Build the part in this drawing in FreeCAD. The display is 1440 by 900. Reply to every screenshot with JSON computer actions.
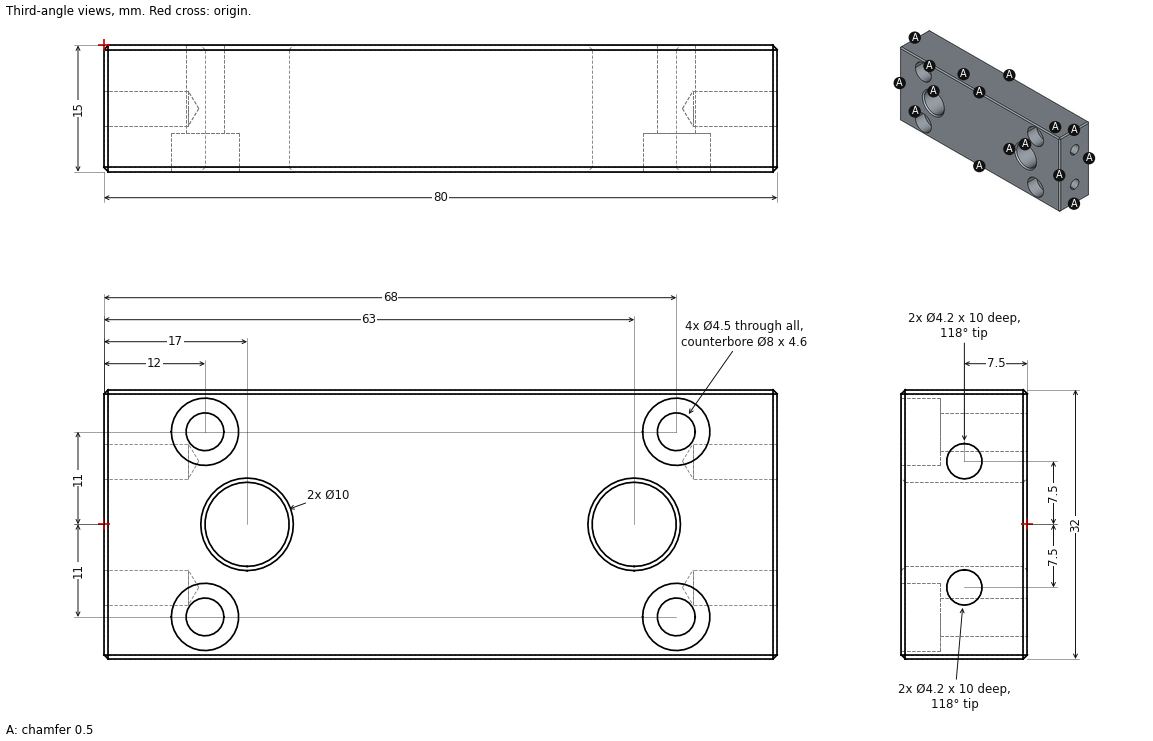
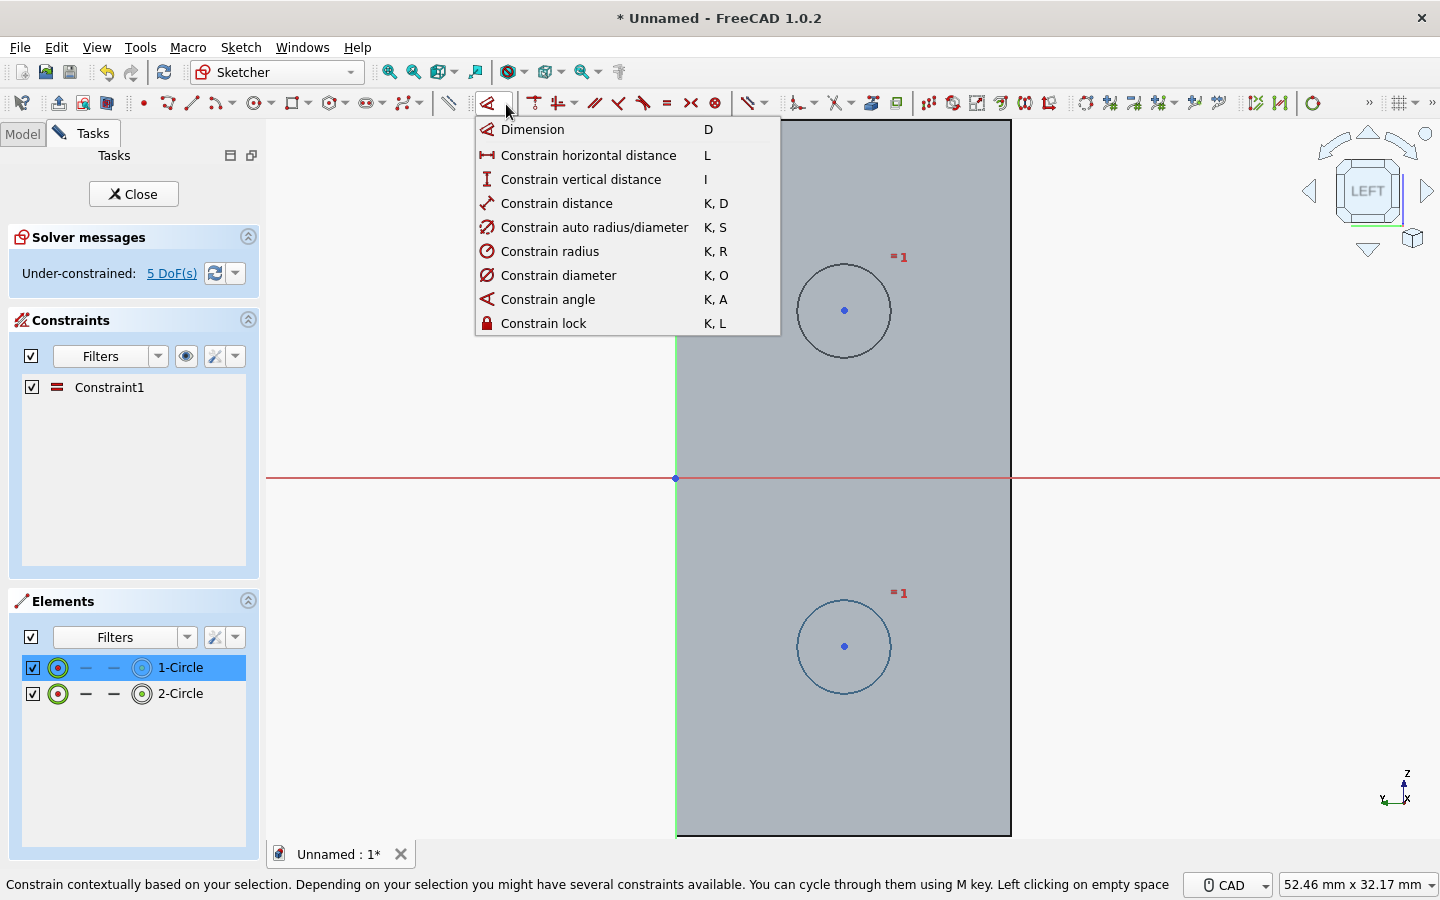
{"action": "left_click", "coordinate": [628, 275]}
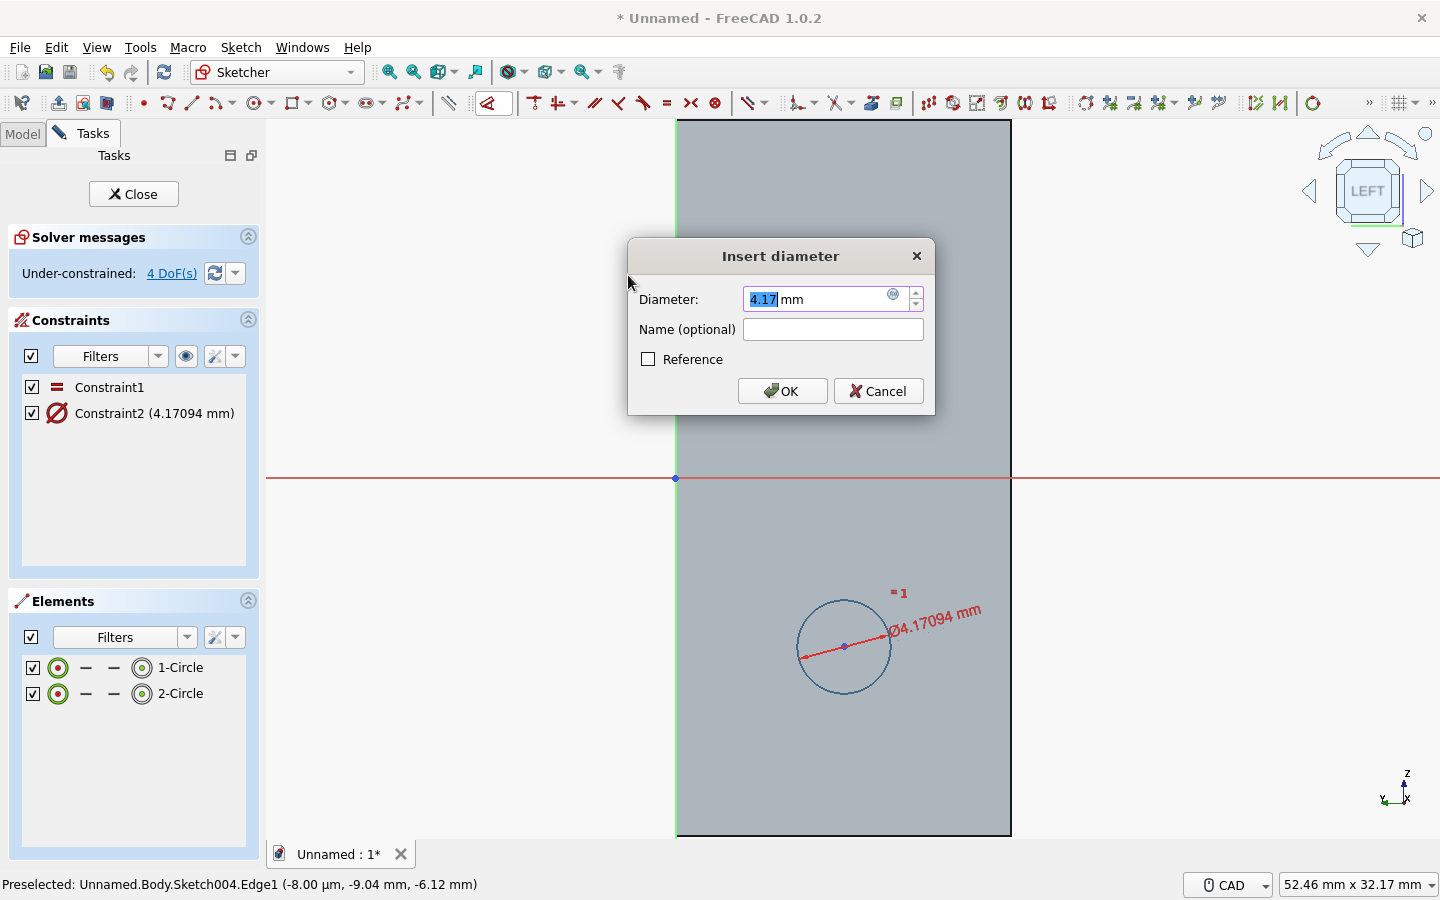
{"action": "type", "text": "4.2"}
{"action": "key", "text": "Return"}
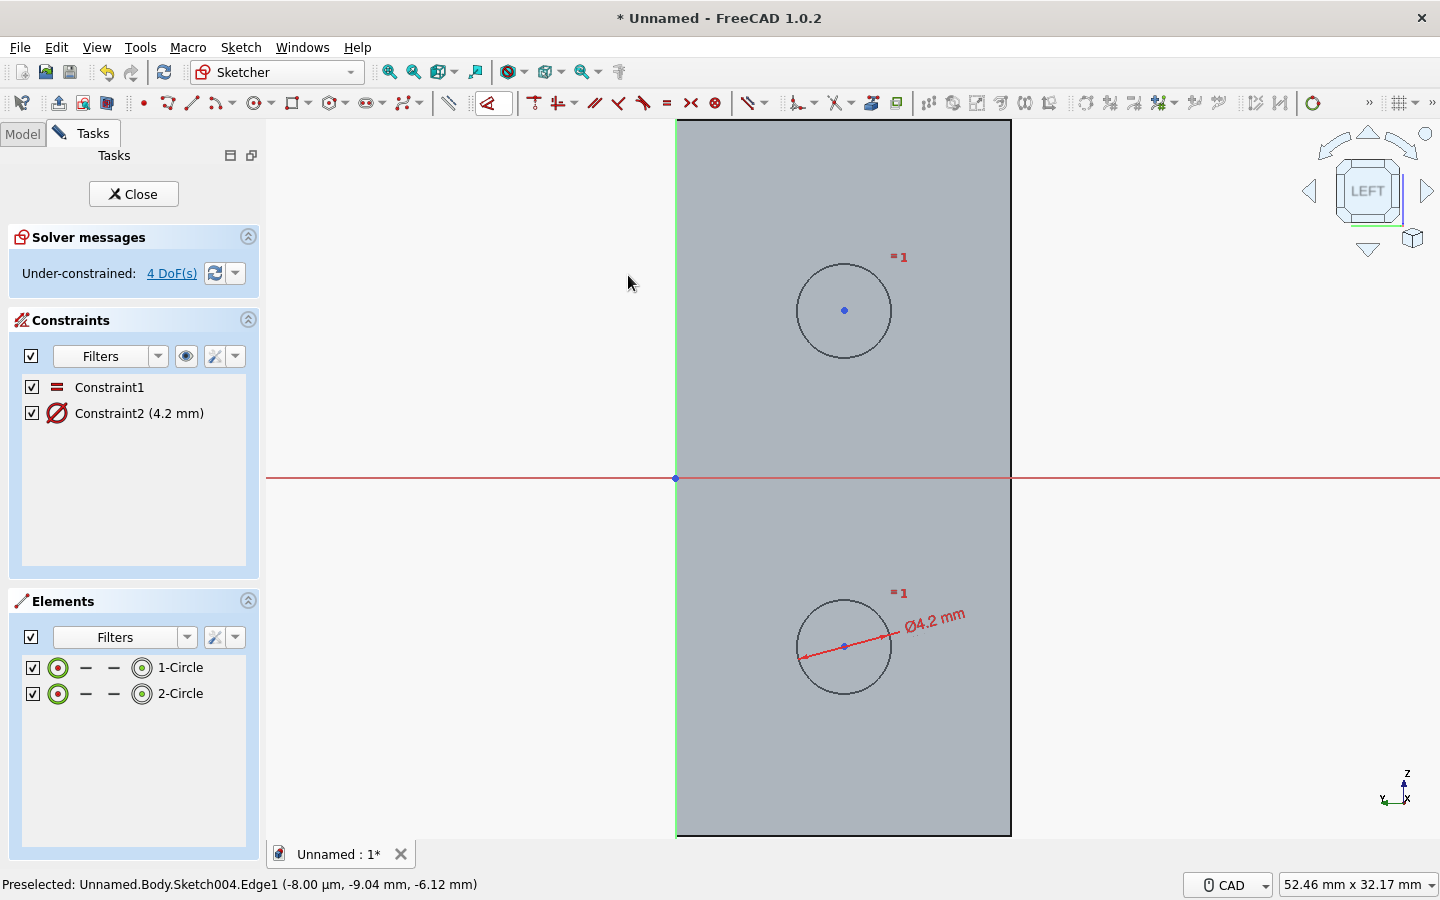
{"action": "left_click", "coordinate": [844, 647]}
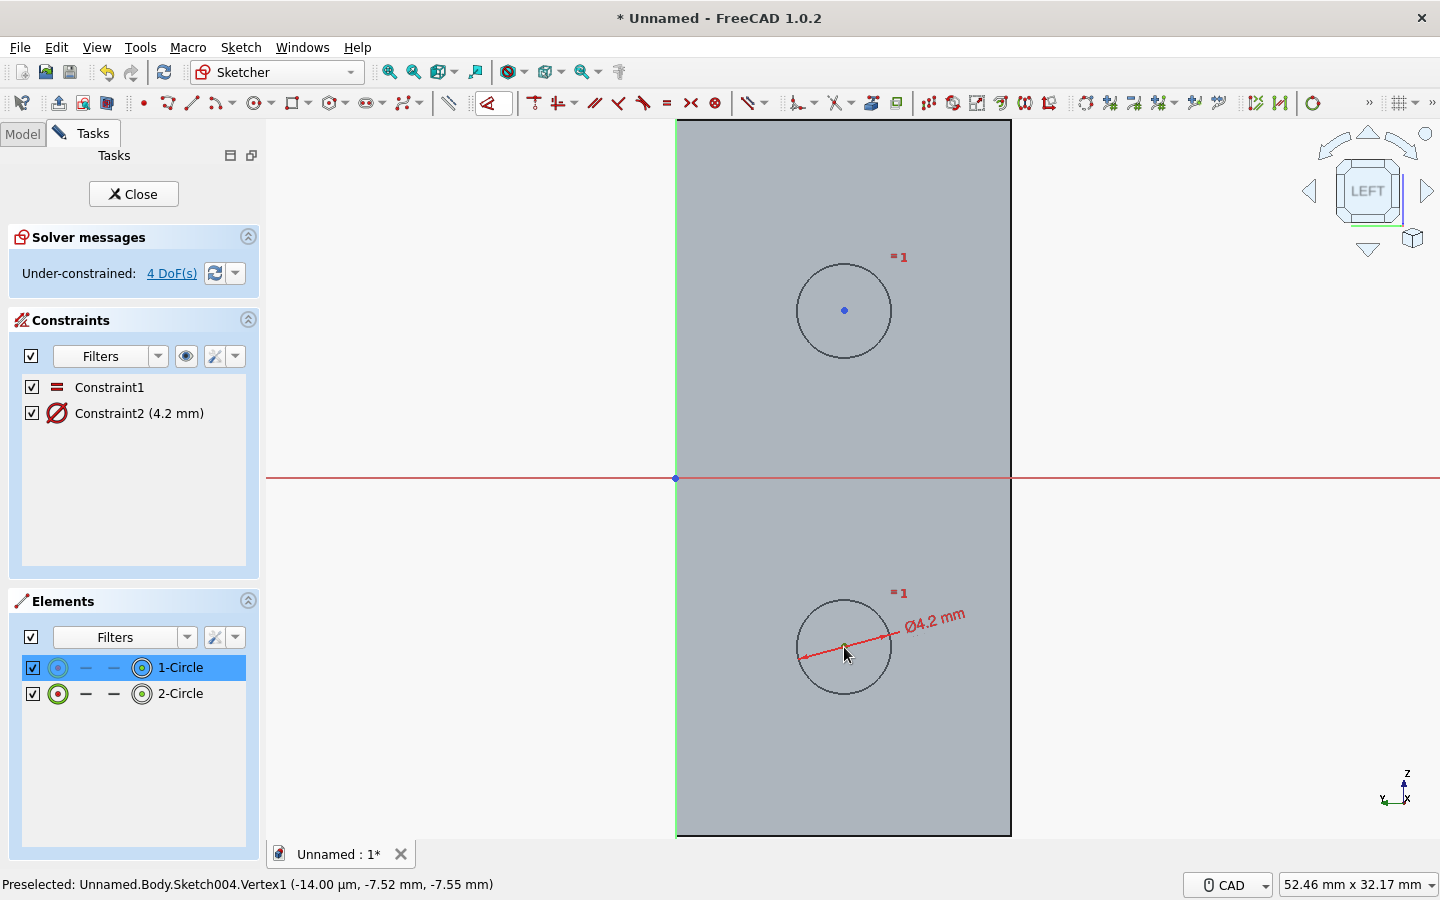
{"action": "left_click", "coordinate": [506, 104]}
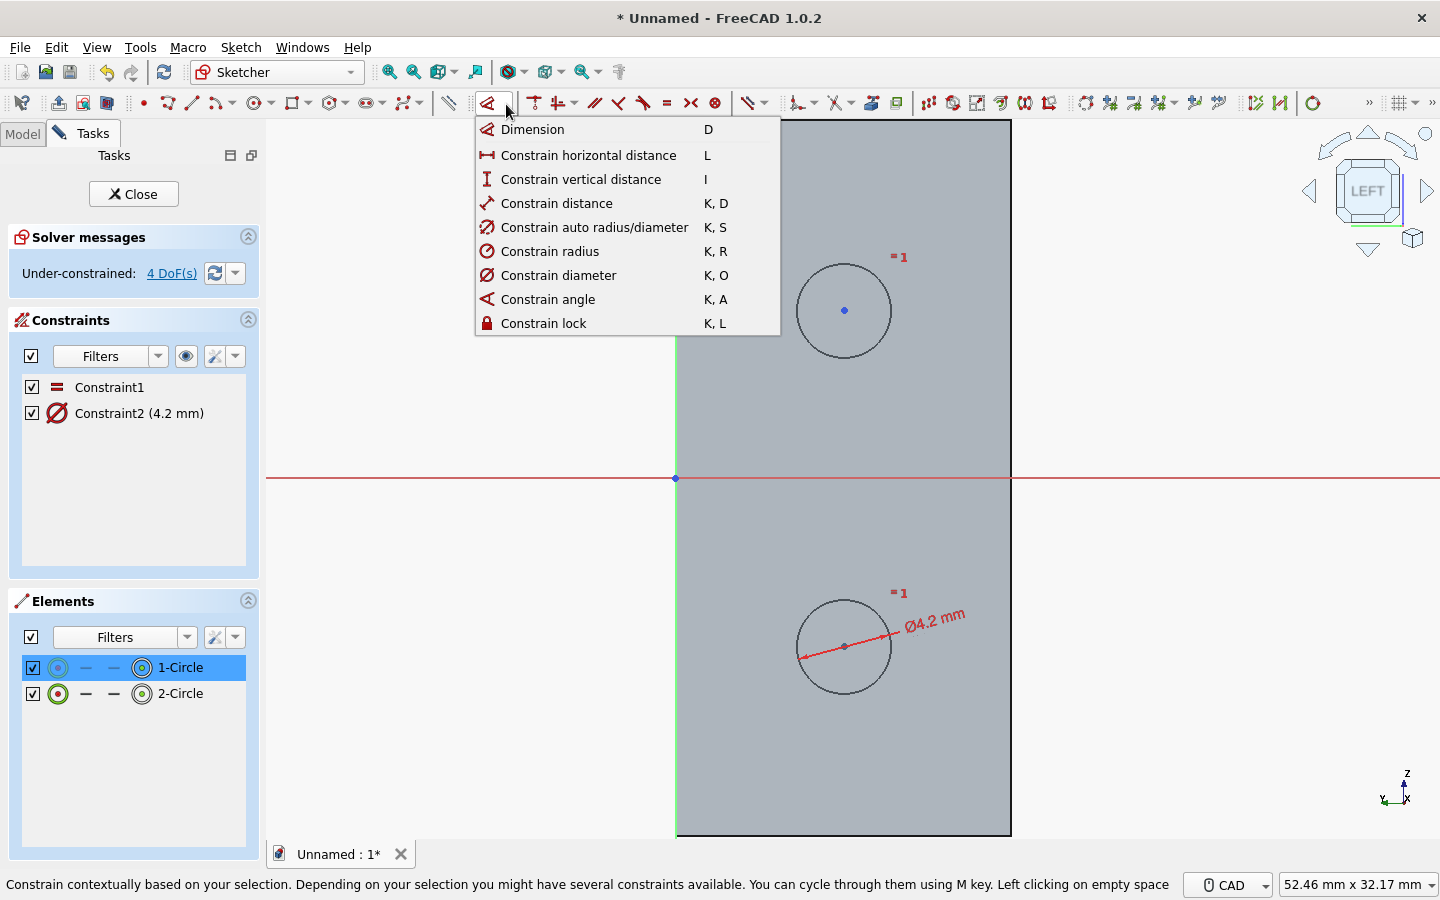
{"action": "left_click", "coordinate": [628, 155]}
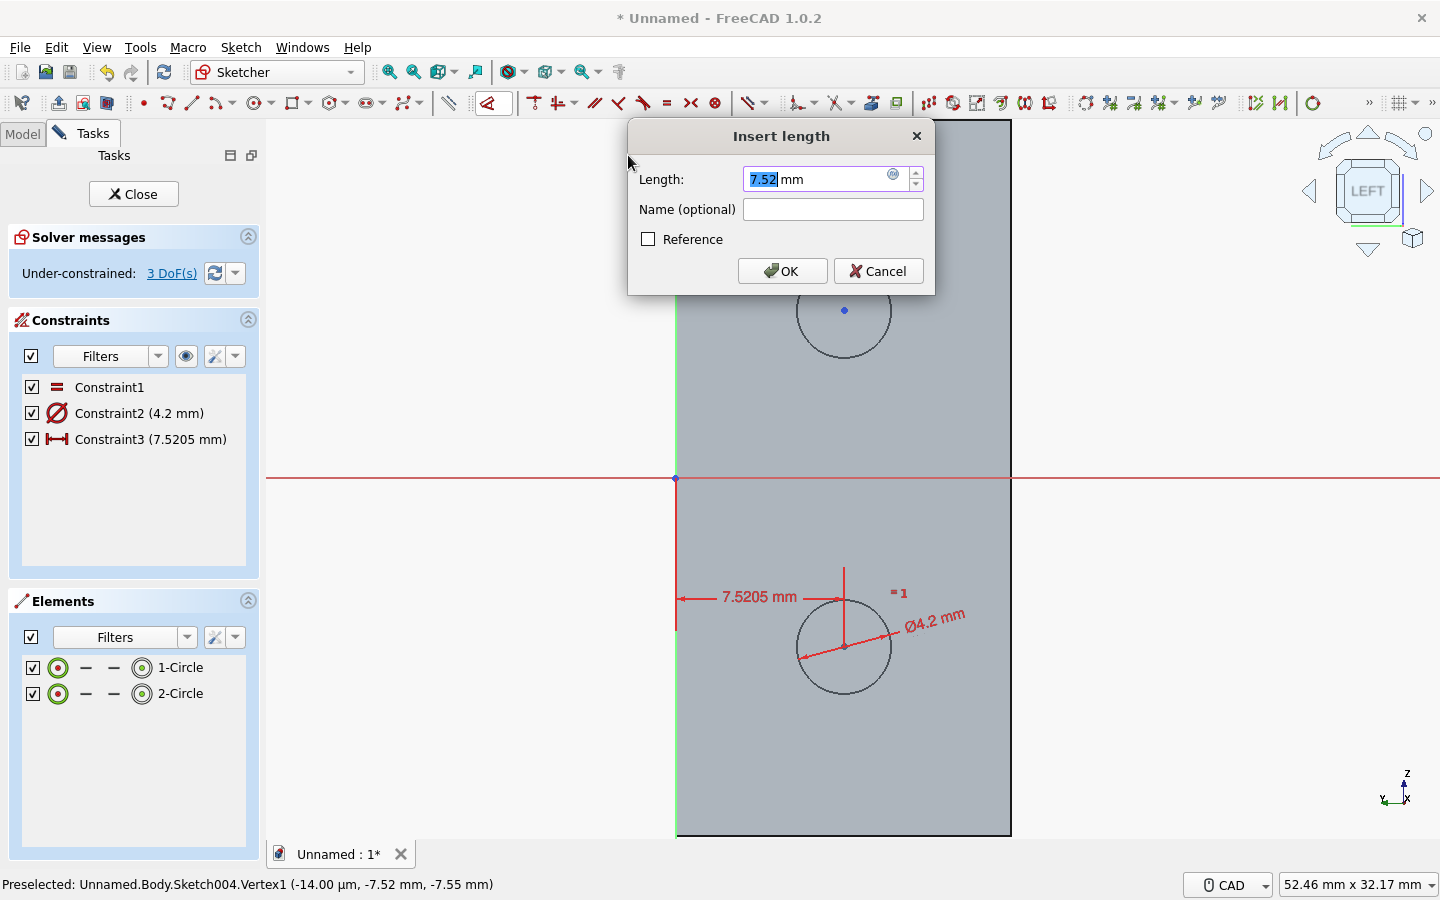
{"action": "type", "text": "7.5"}
{"action": "key", "text": "Return"}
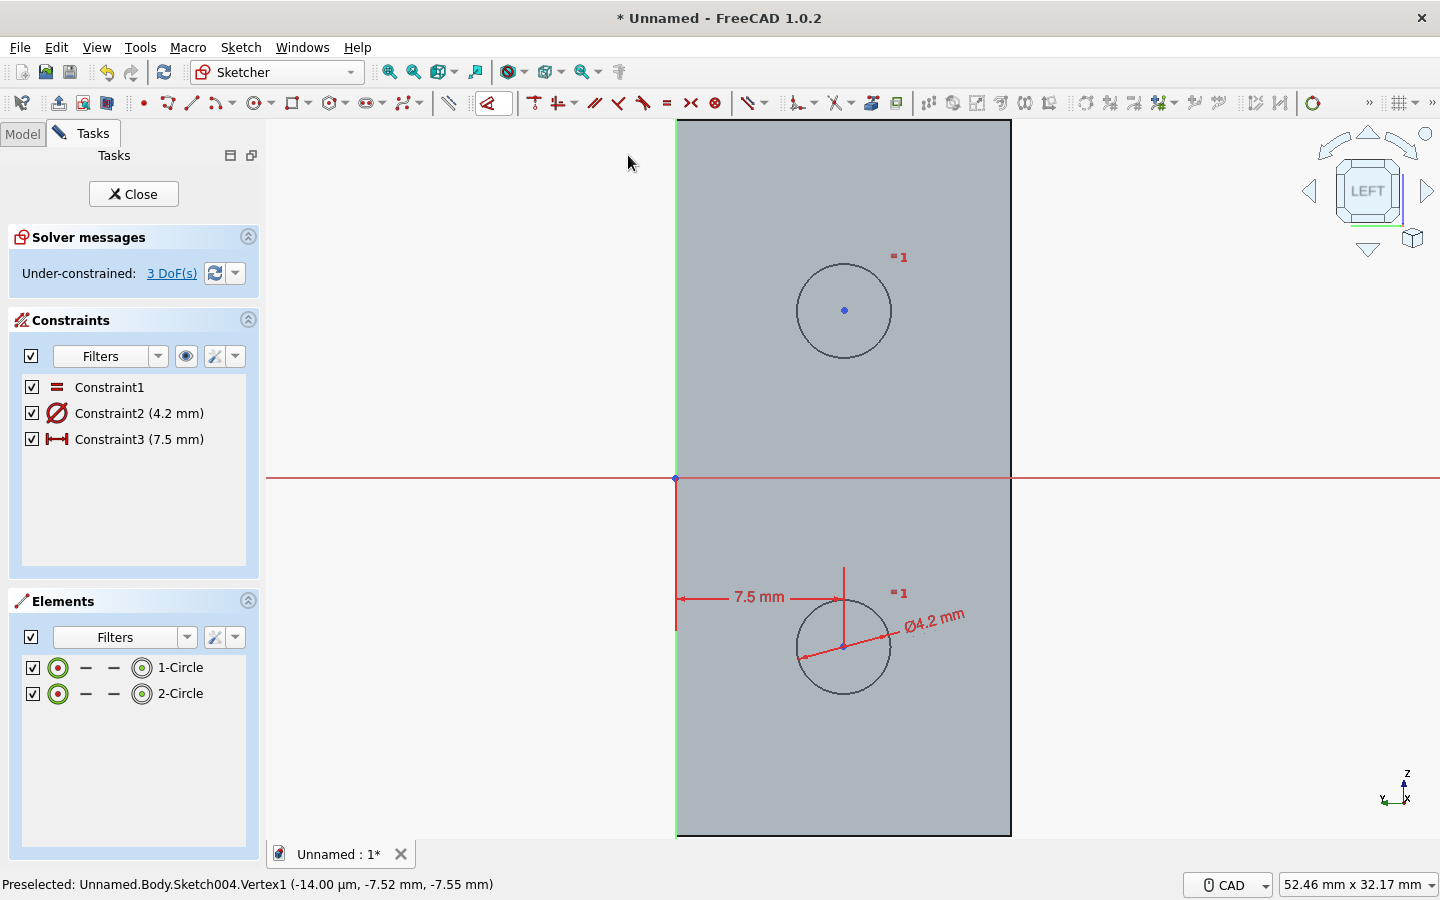
{"action": "left_click", "coordinate": [844, 647]}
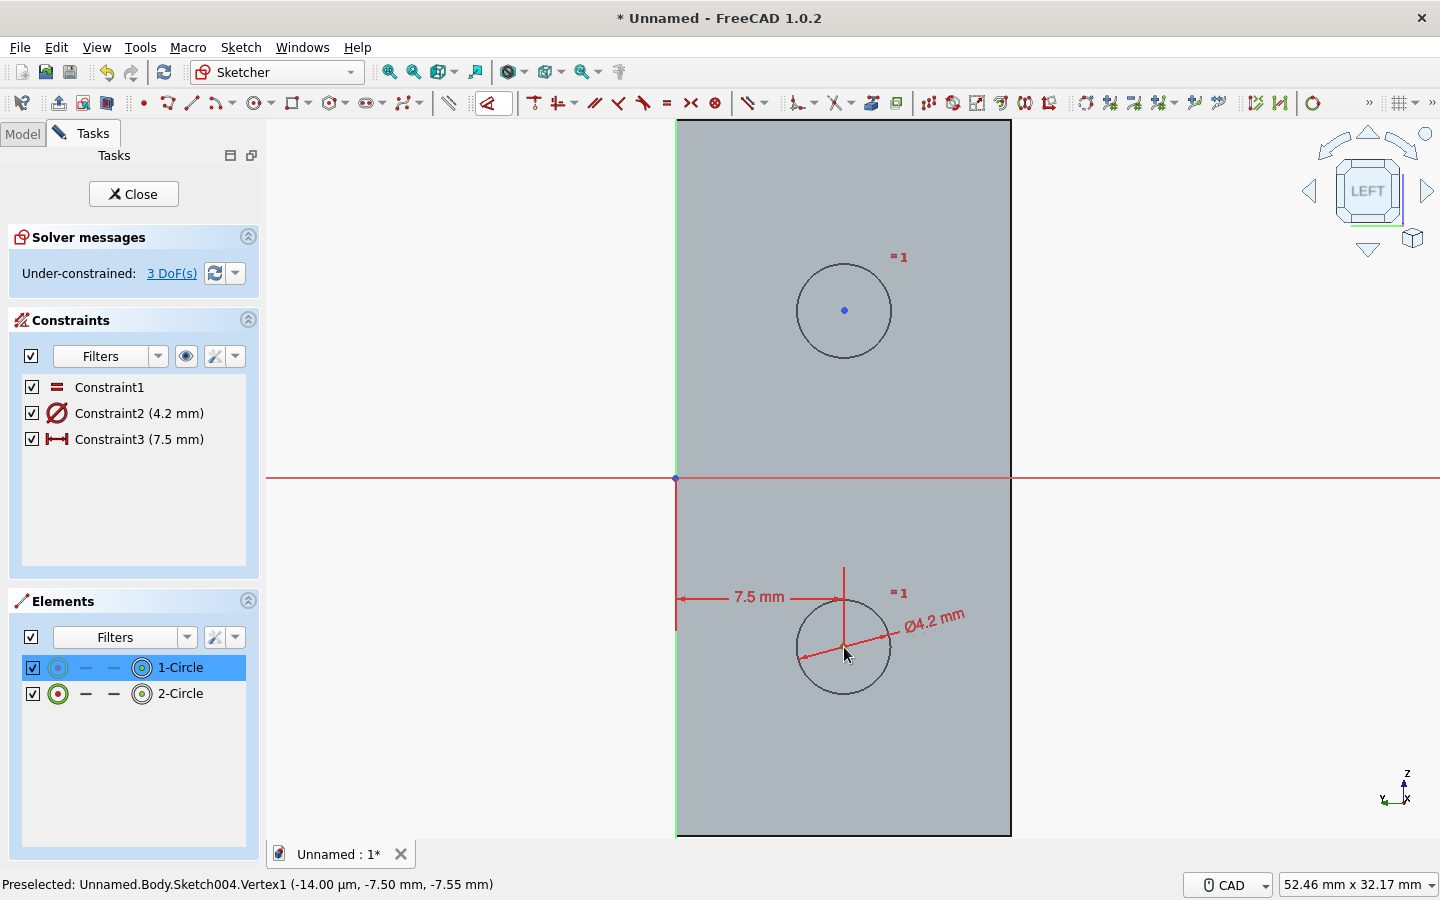
{"action": "left_click", "coordinate": [506, 104]}